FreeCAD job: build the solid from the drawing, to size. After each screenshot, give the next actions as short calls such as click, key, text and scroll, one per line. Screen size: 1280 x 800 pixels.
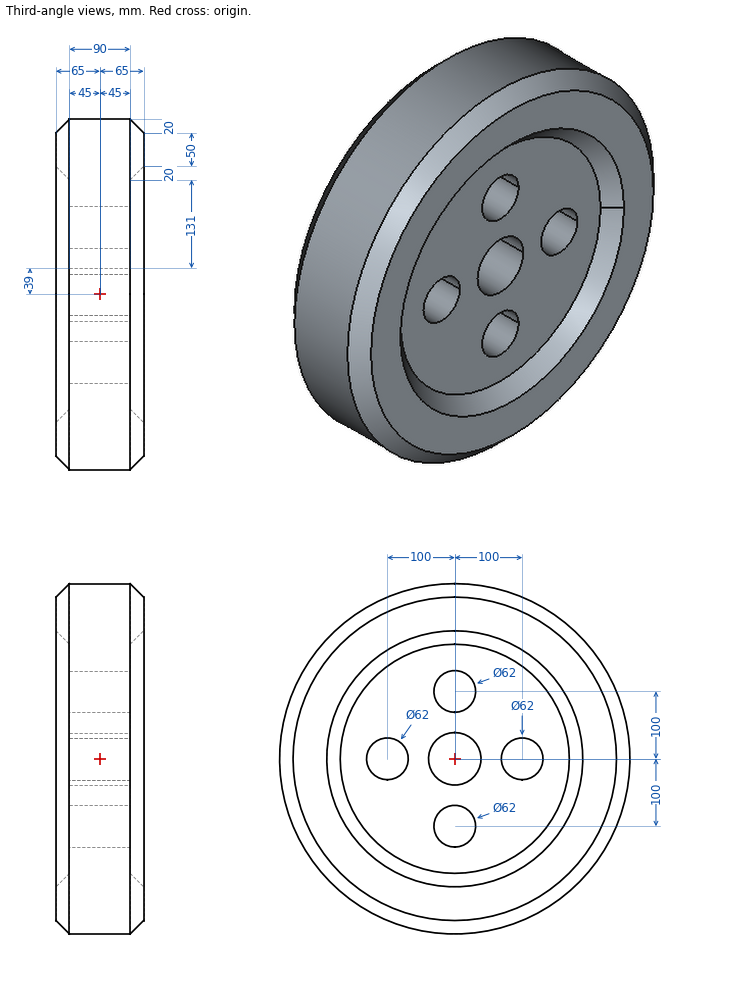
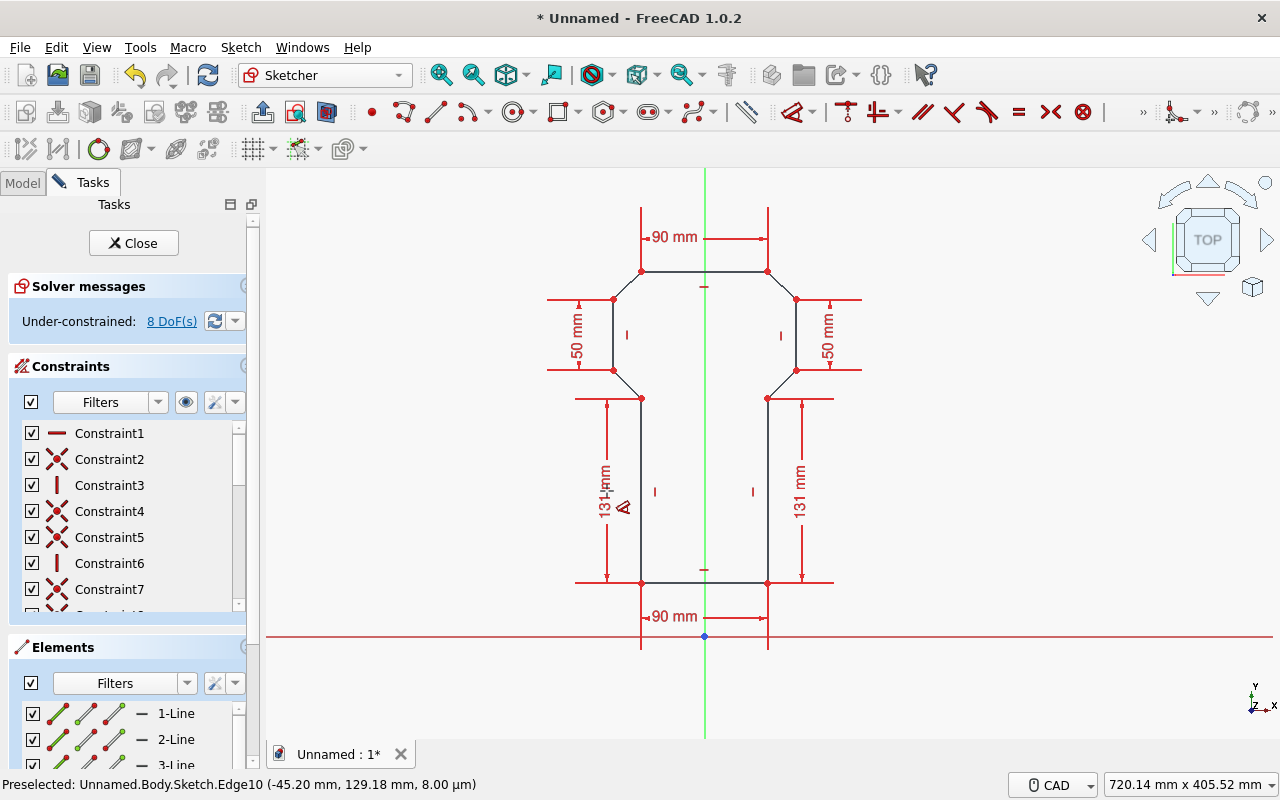
click(641, 583)
click(673, 671)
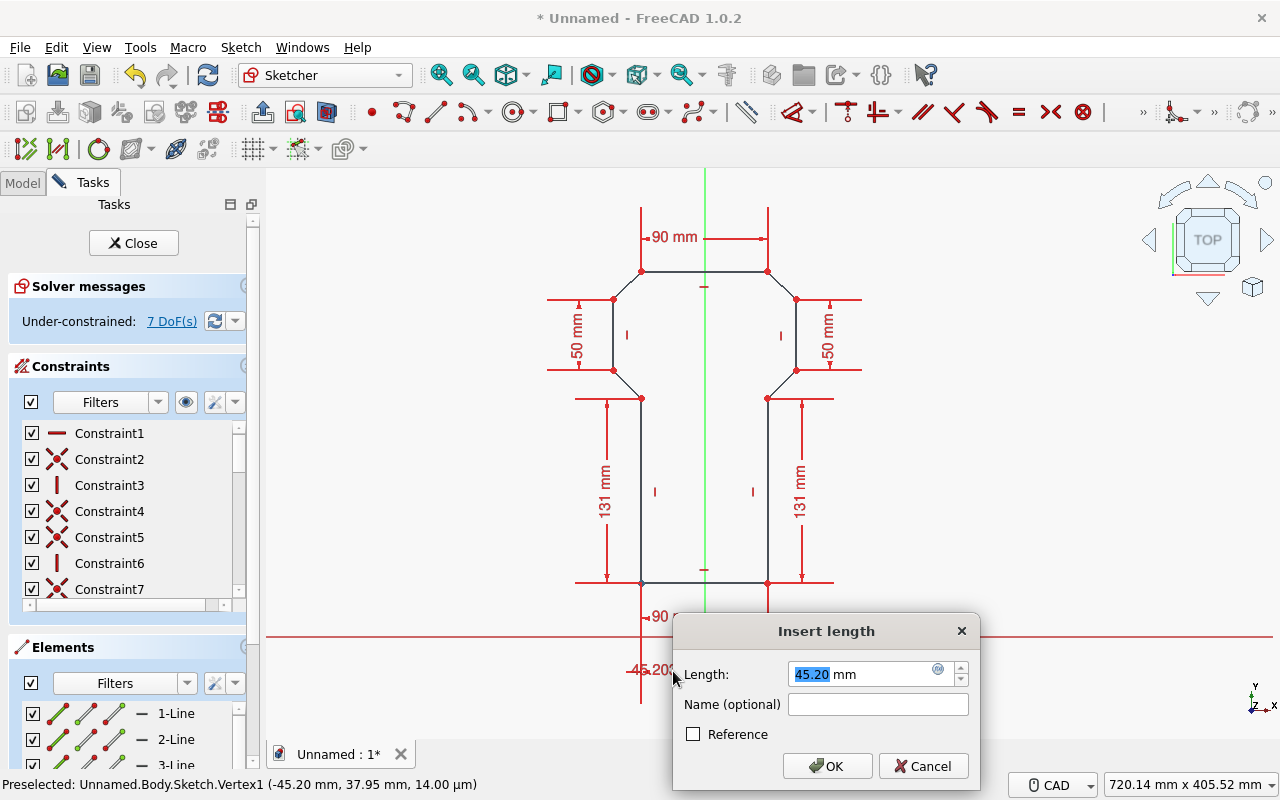
text(45)
key(Return)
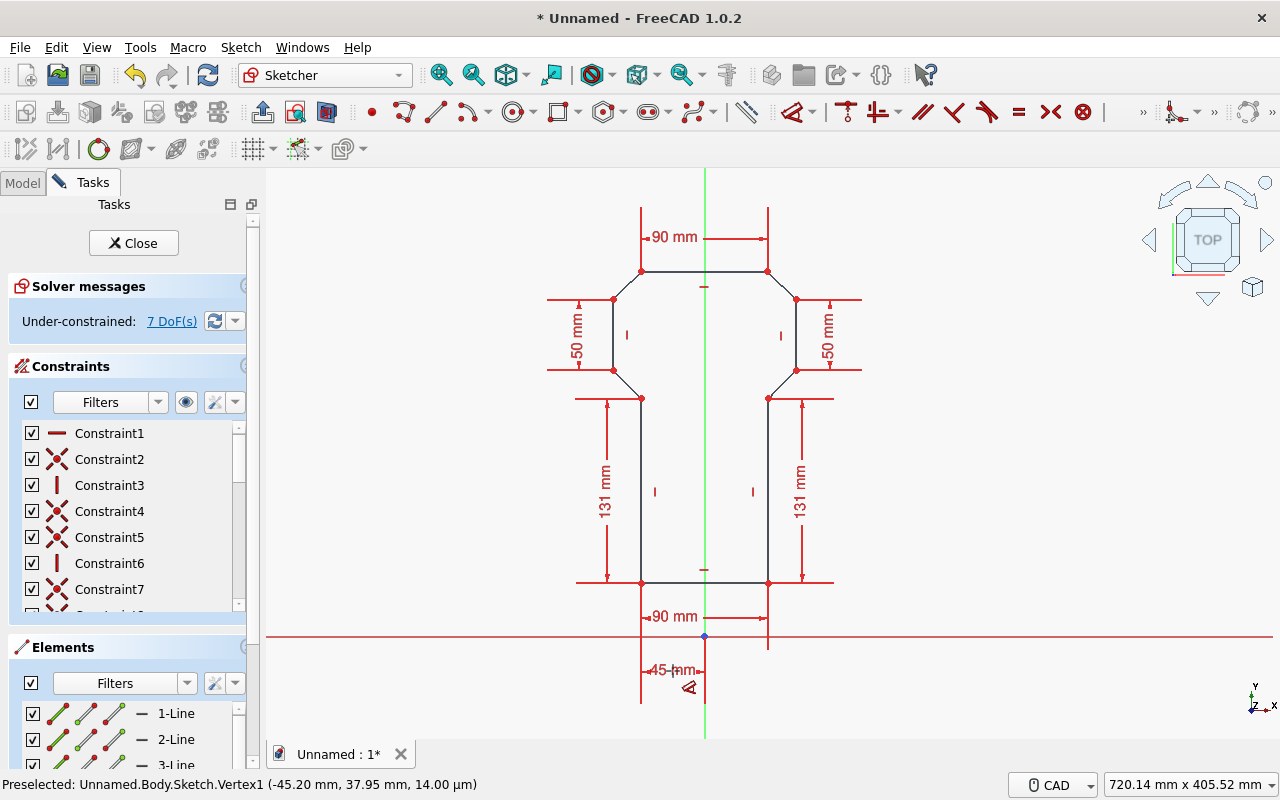
click(641, 583)
click(607, 591)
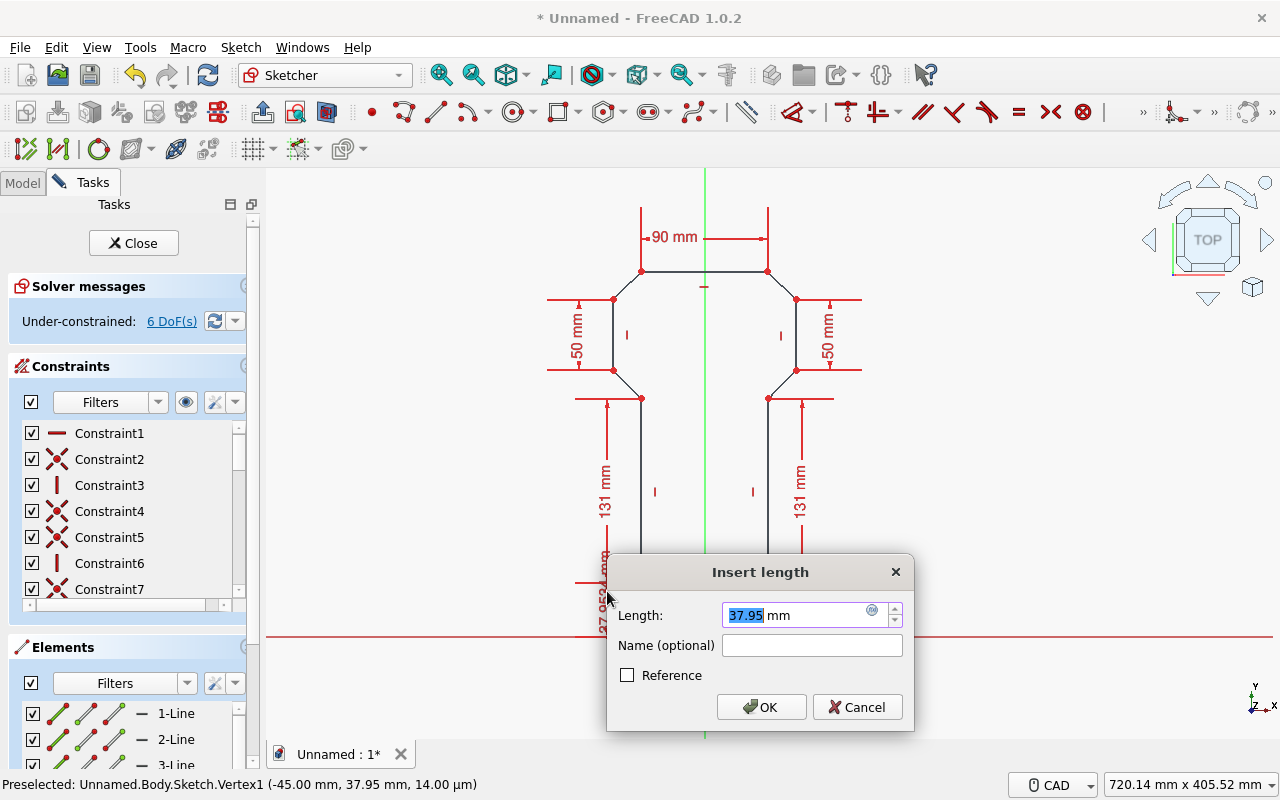
text(39)
key(Return)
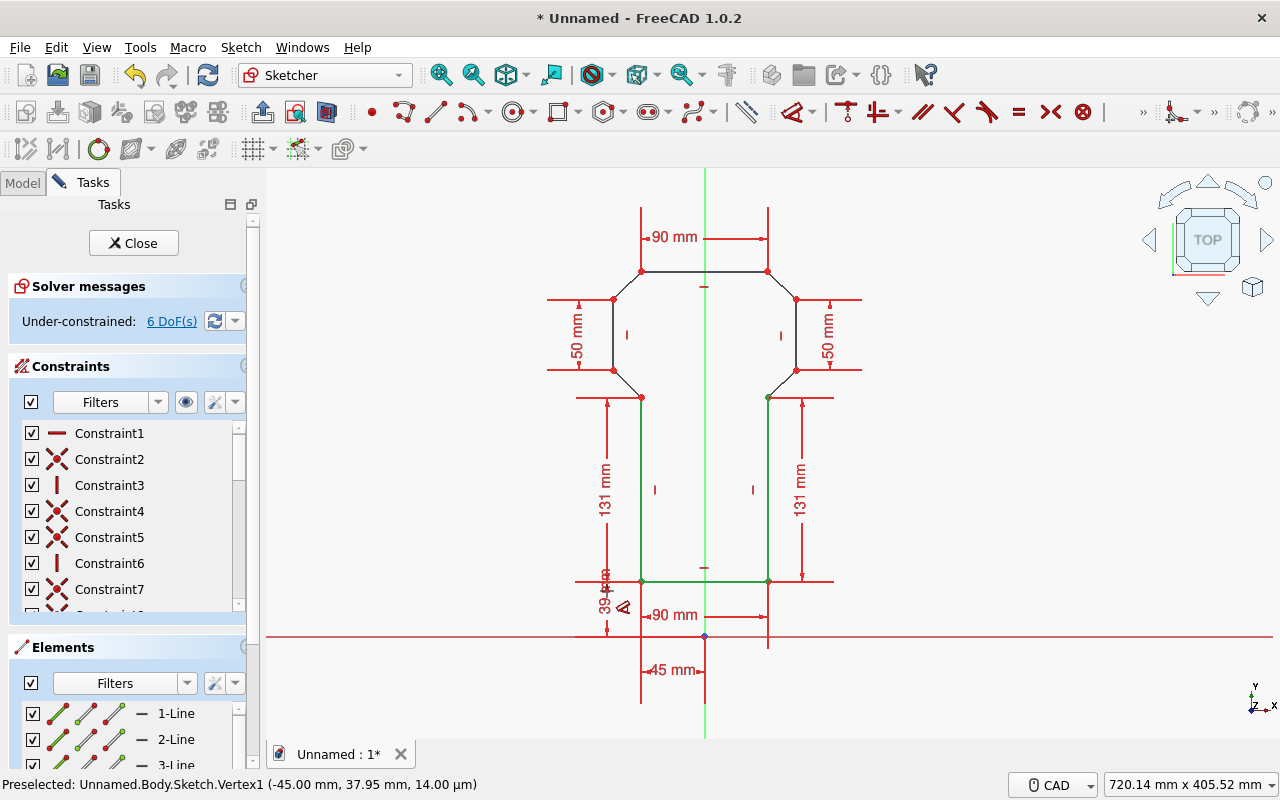
click(796, 370)
click(750, 671)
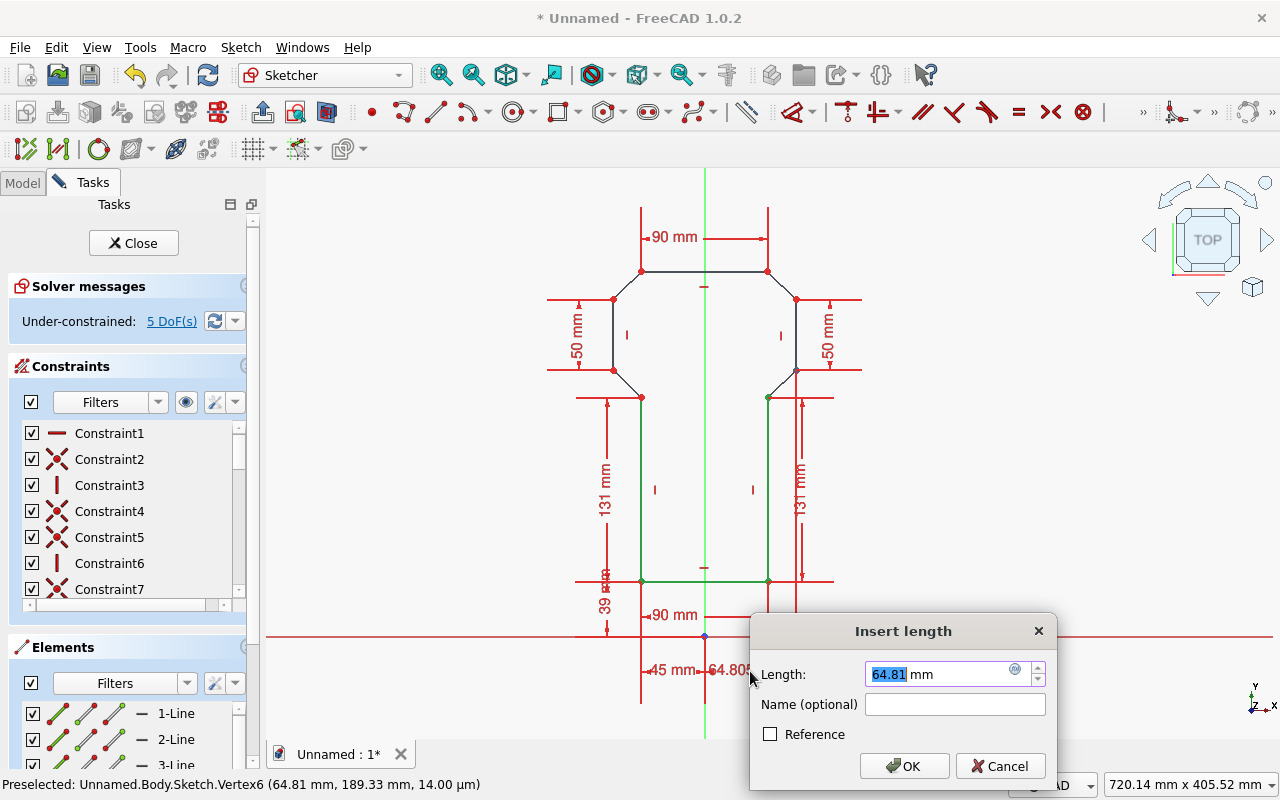
text(65)
key(Return)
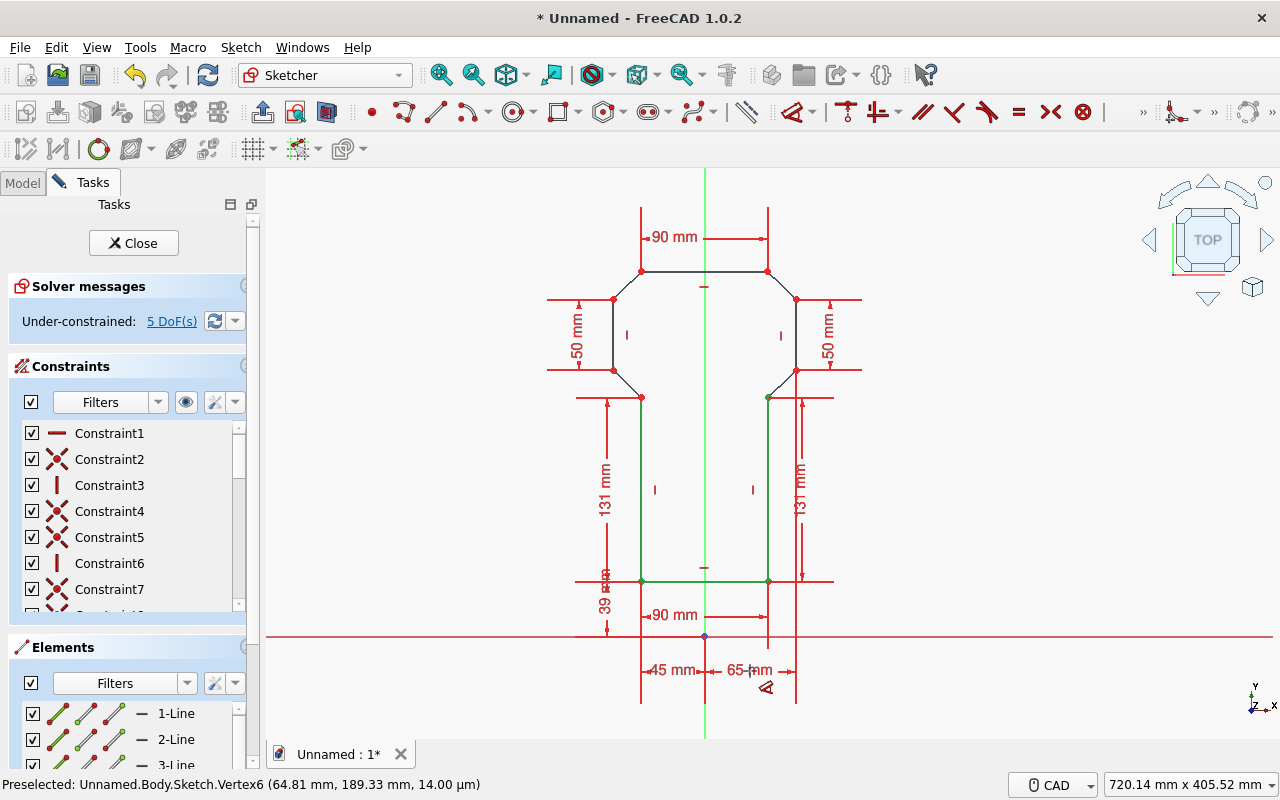
click(768, 272)
click(751, 238)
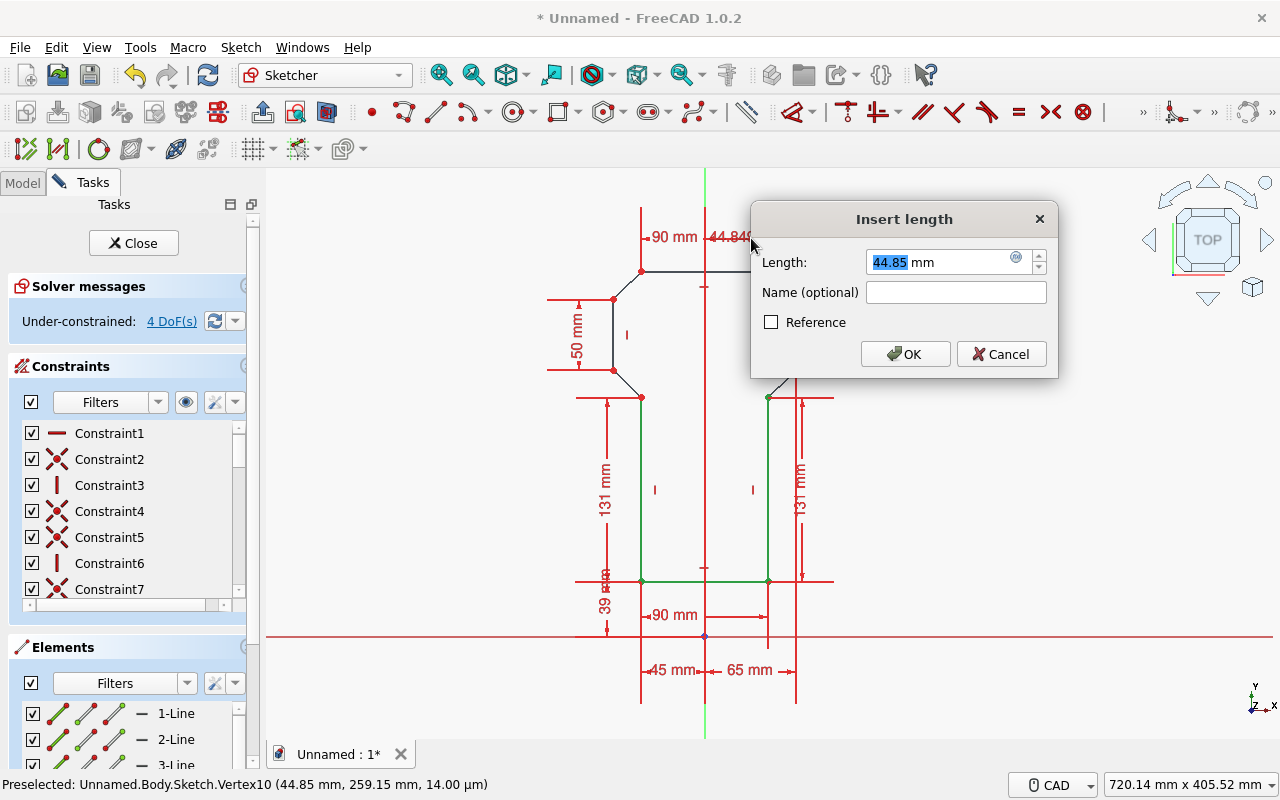
text(45)
key(Return)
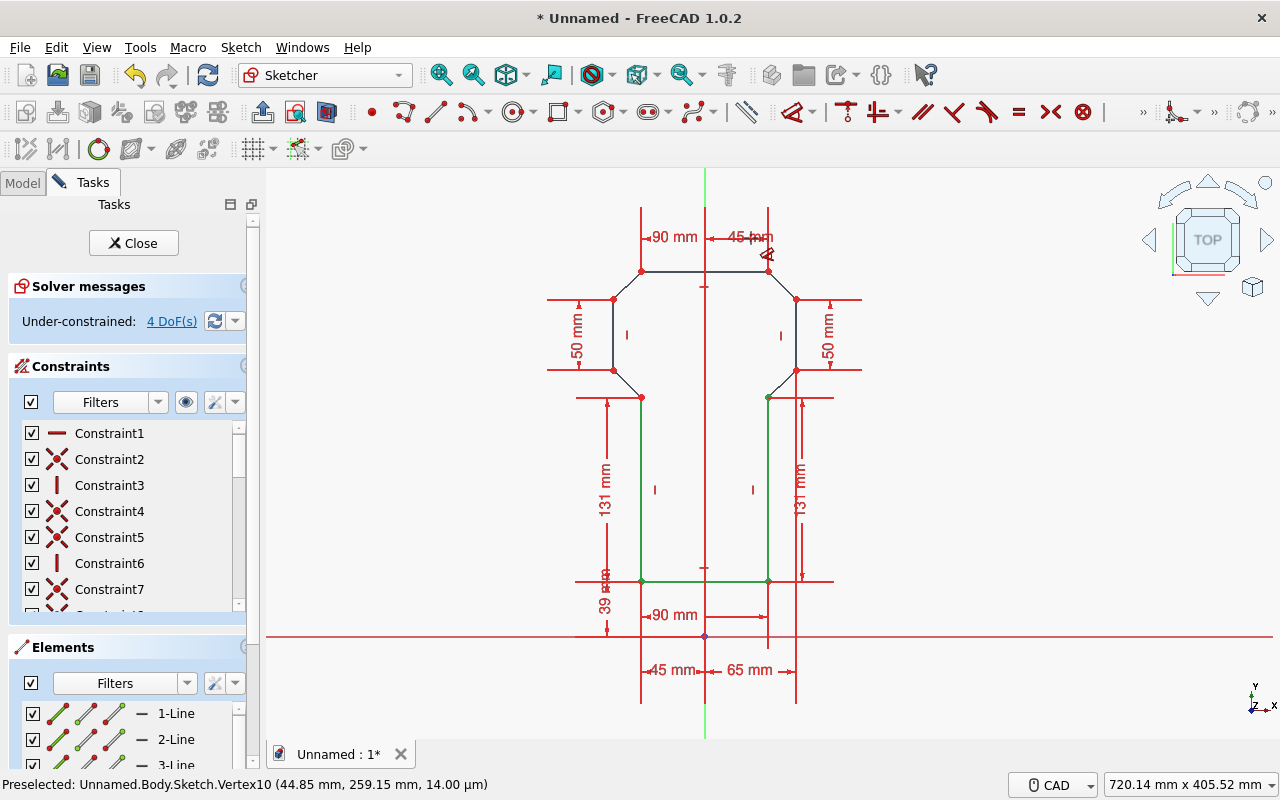
click(613, 300)
click(627, 266)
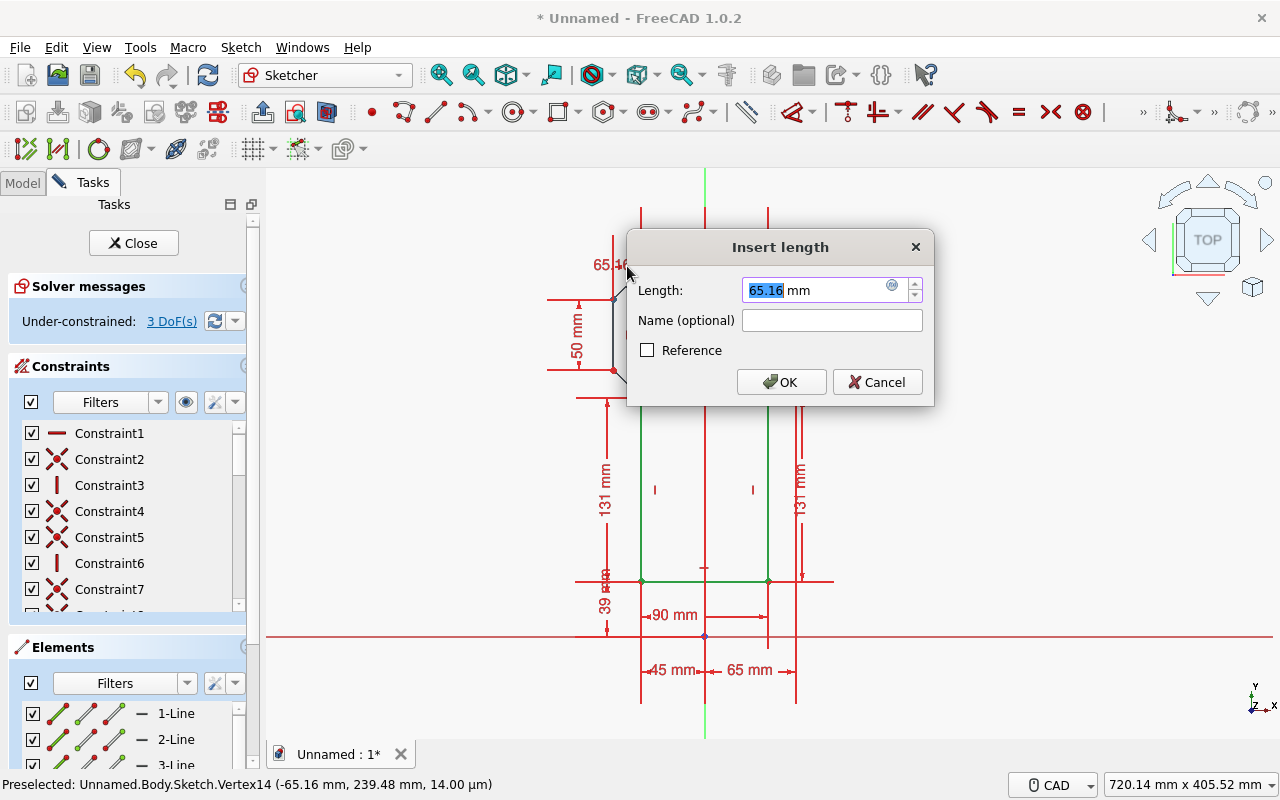
text(65)
key(Return)